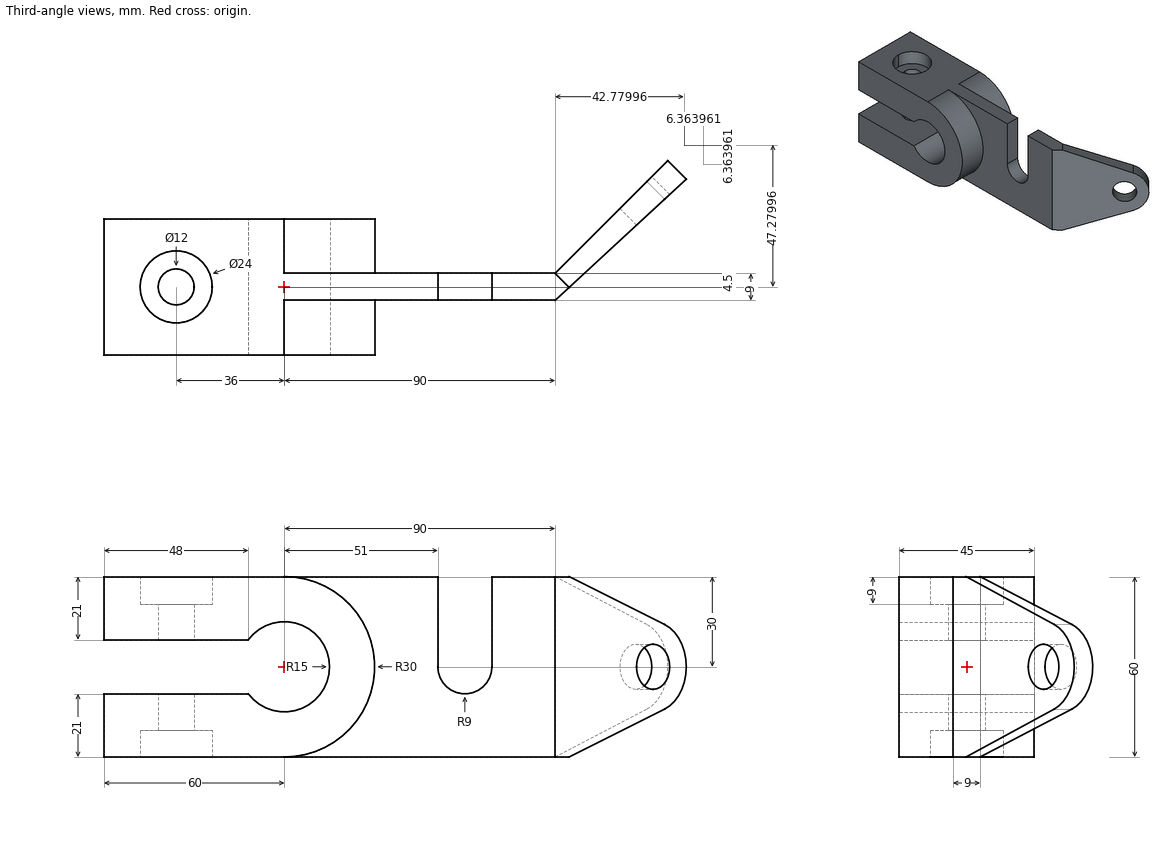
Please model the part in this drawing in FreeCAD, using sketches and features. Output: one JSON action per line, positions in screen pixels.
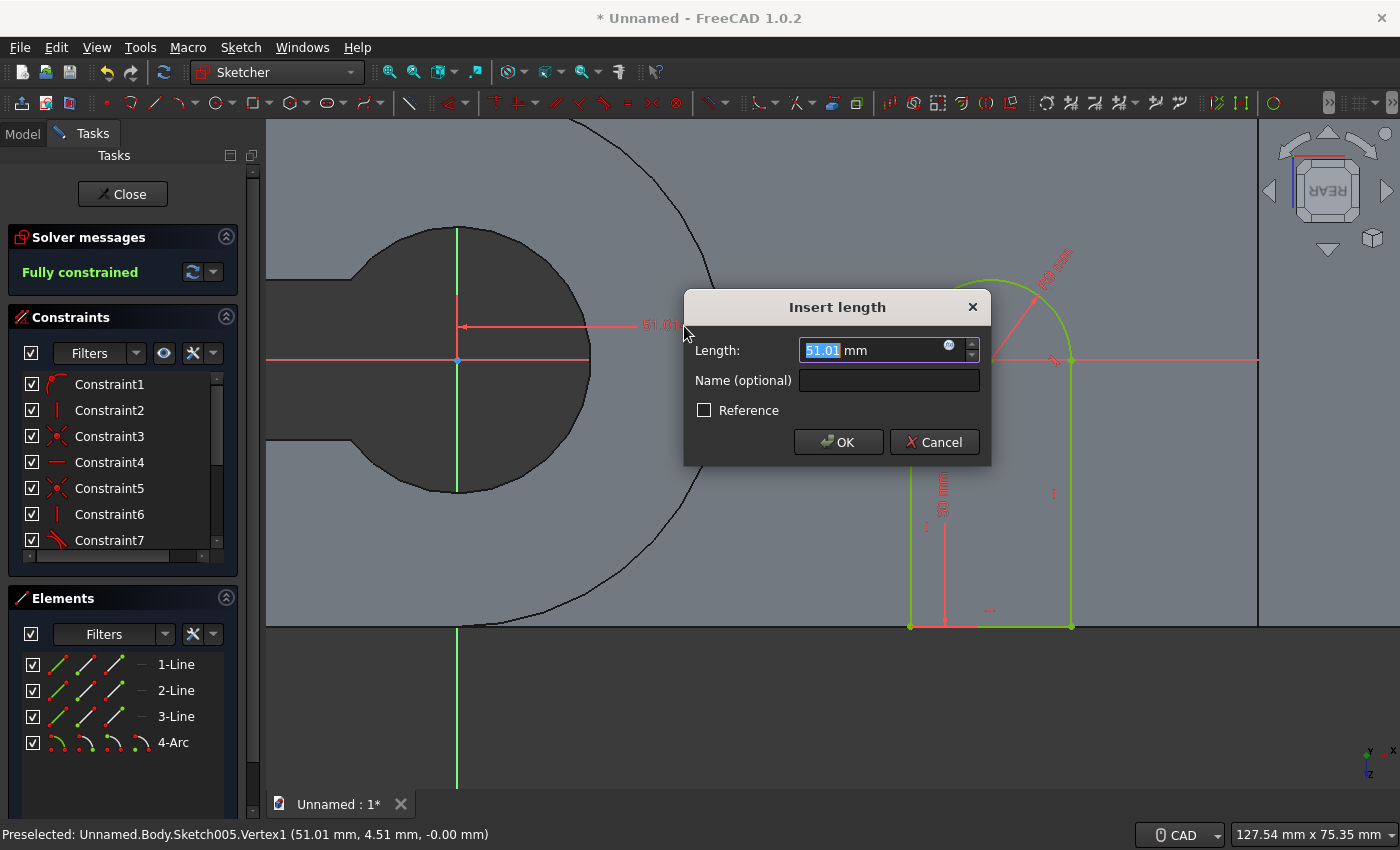
{"action": "type", "text": "51"}
{"action": "key", "text": "Return"}
{"action": "key", "text": "Escape"}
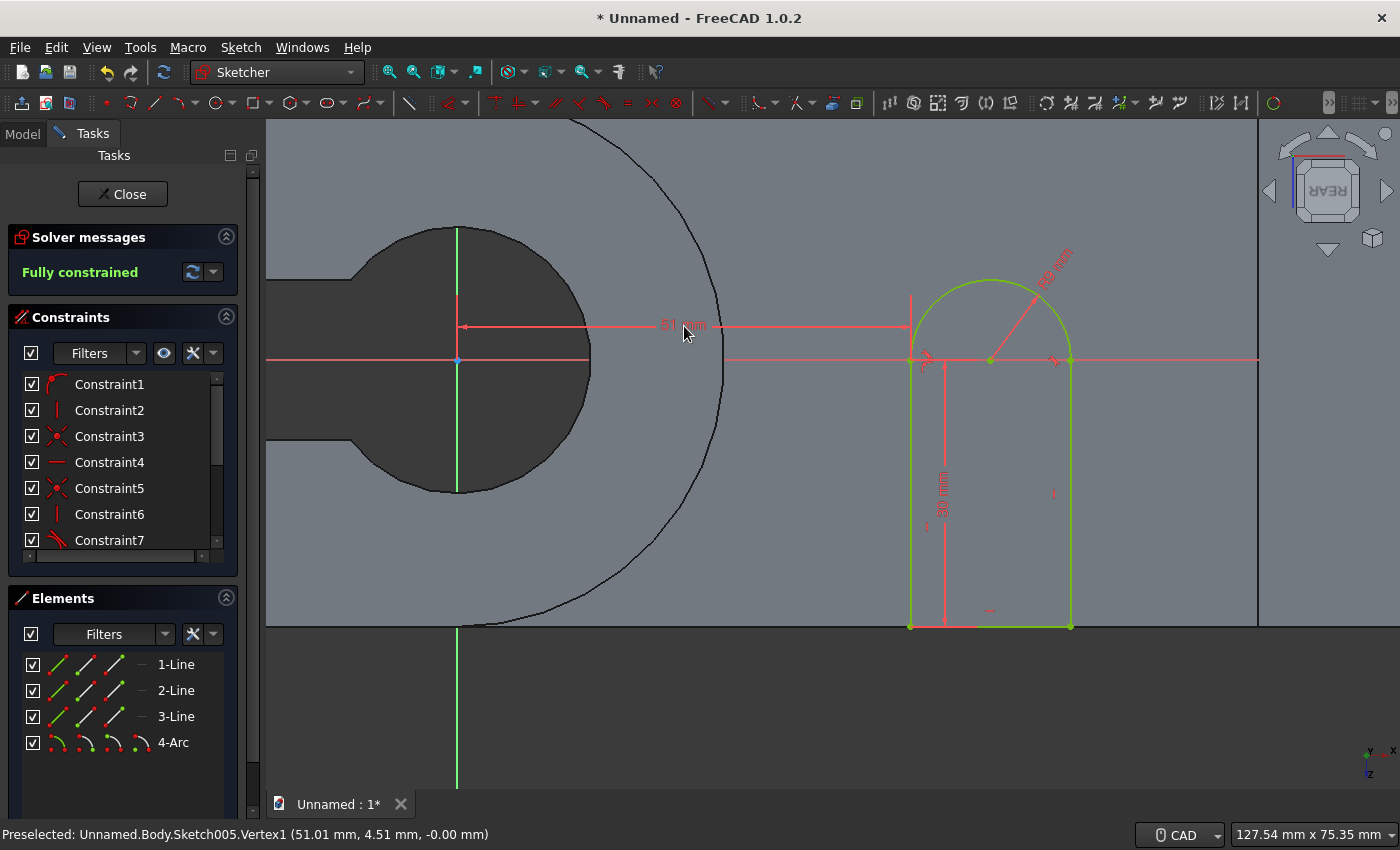
{"action": "left_click", "coordinate": [123, 194]}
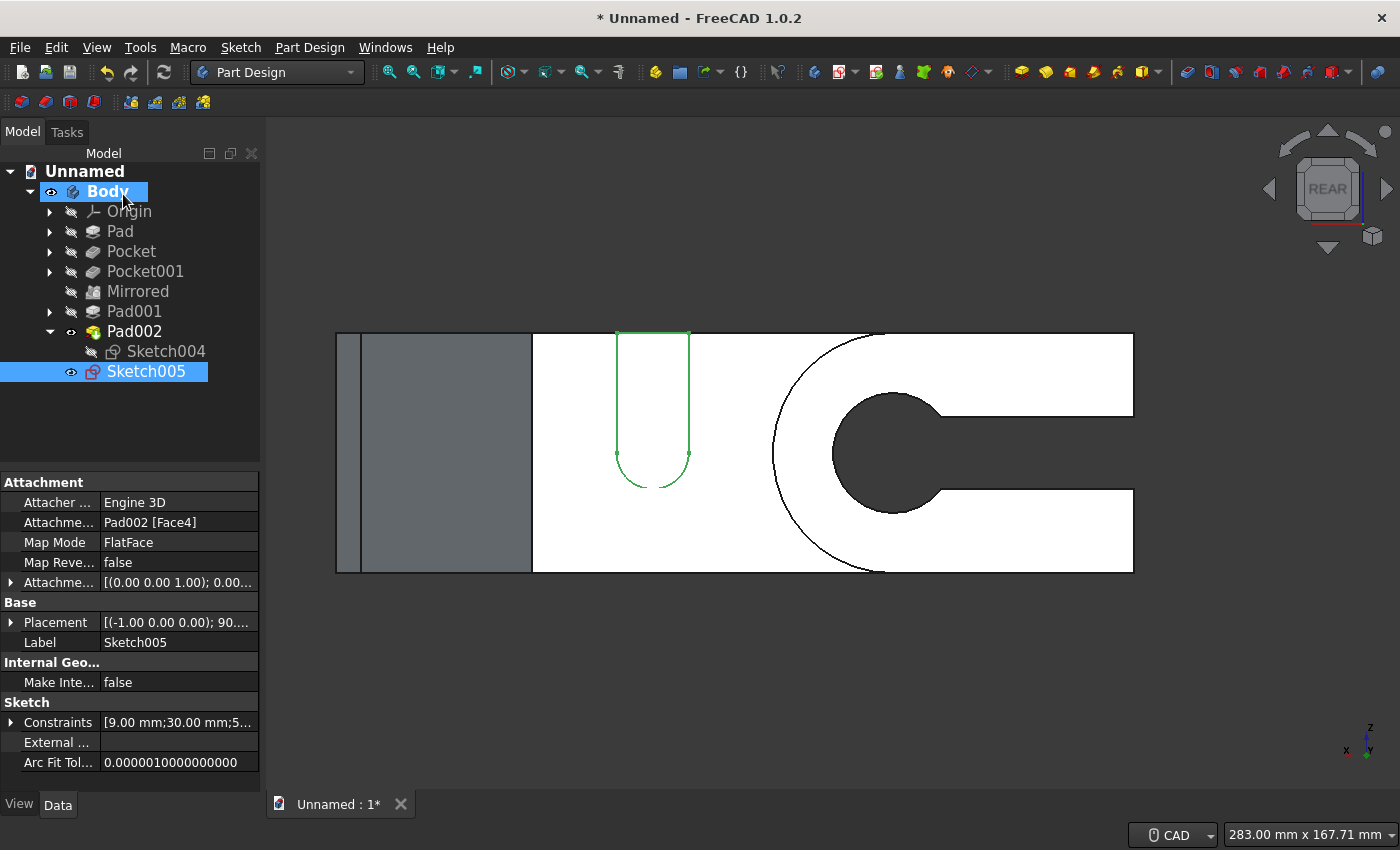
{"action": "left_click", "coordinate": [1188, 72]}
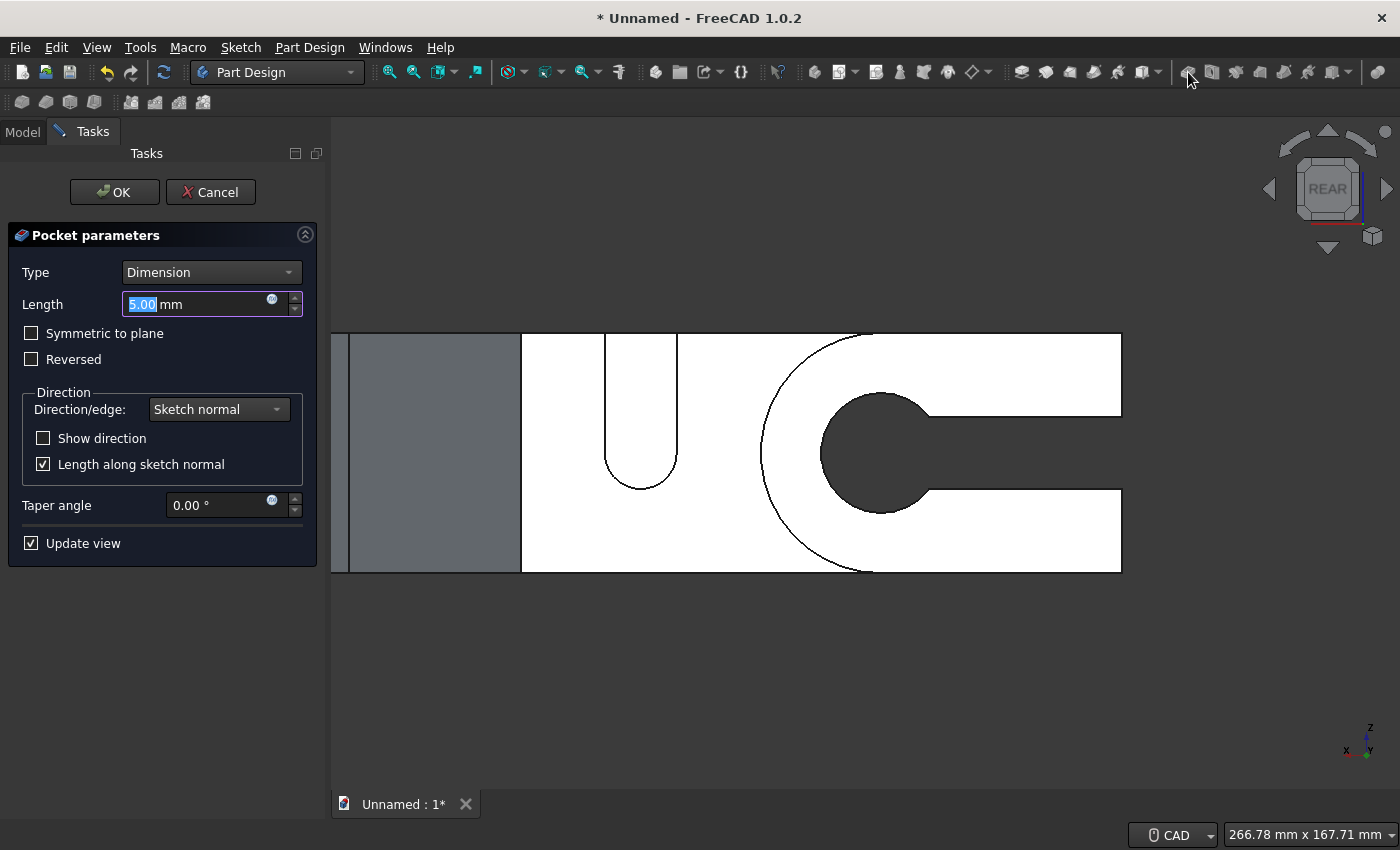
{"action": "type", "text": "9"}
{"action": "key", "text": "Tab"}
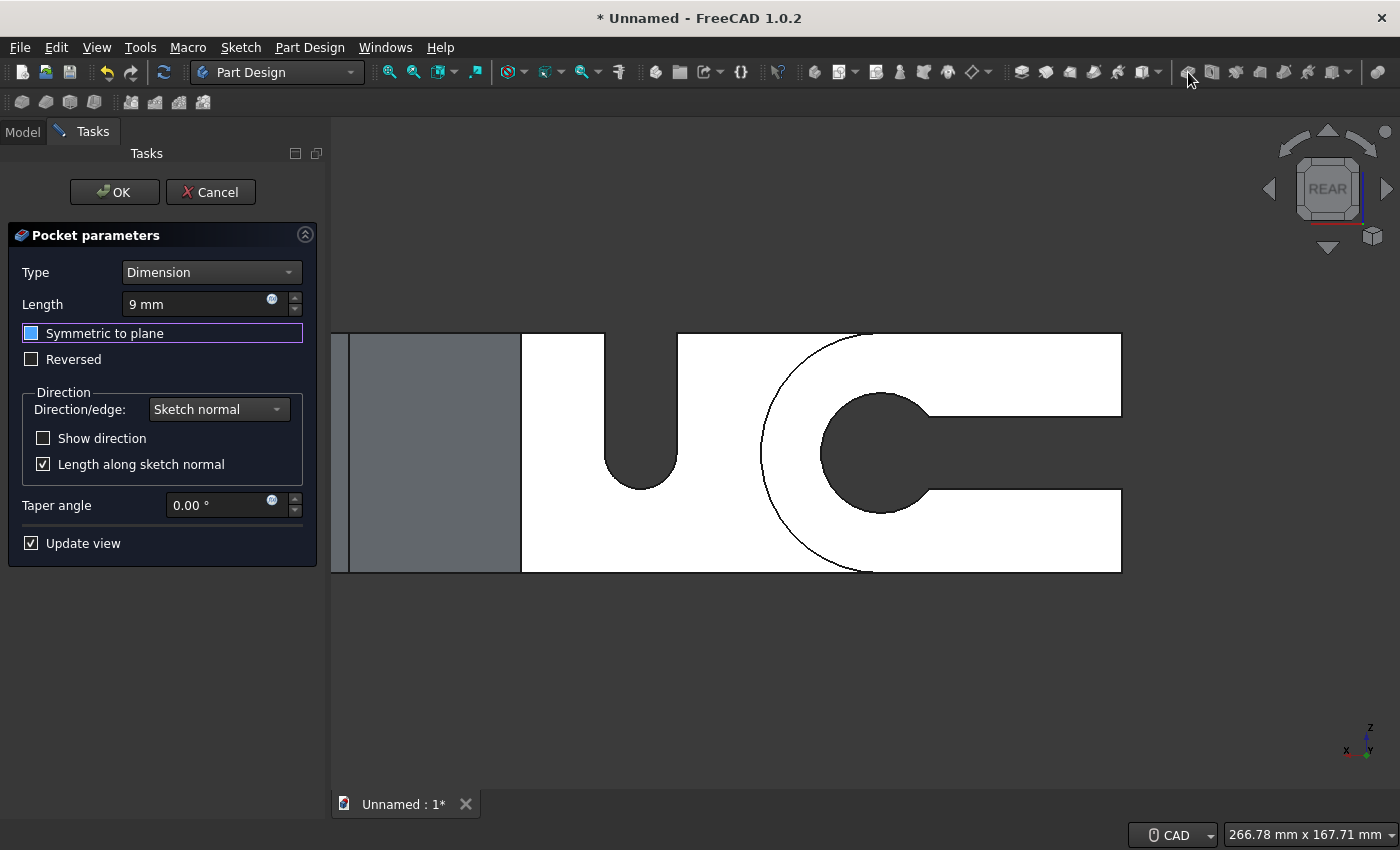
{"action": "left_click", "coordinate": [115, 192]}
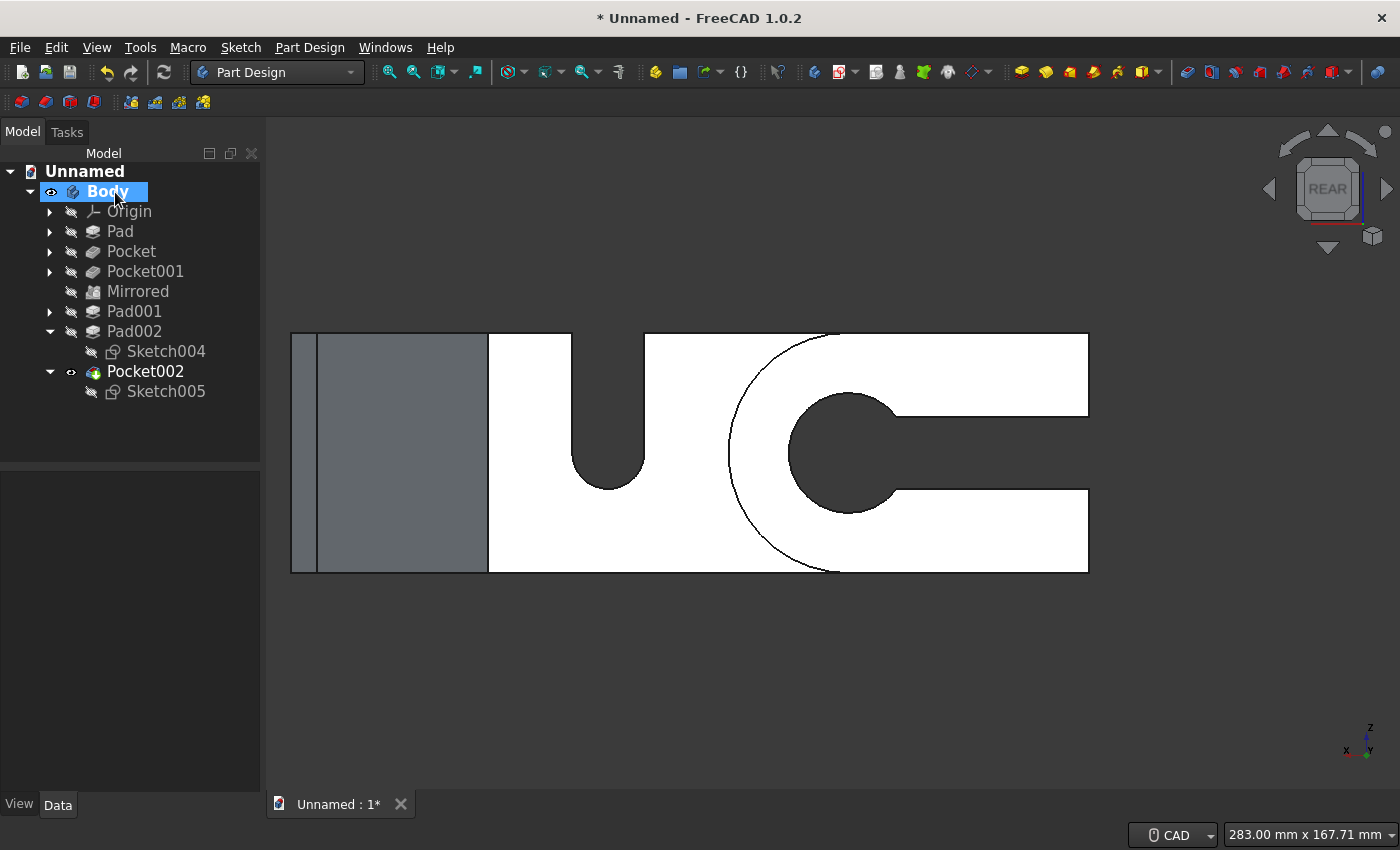
{"action": "left_click", "coordinate": [402, 452]}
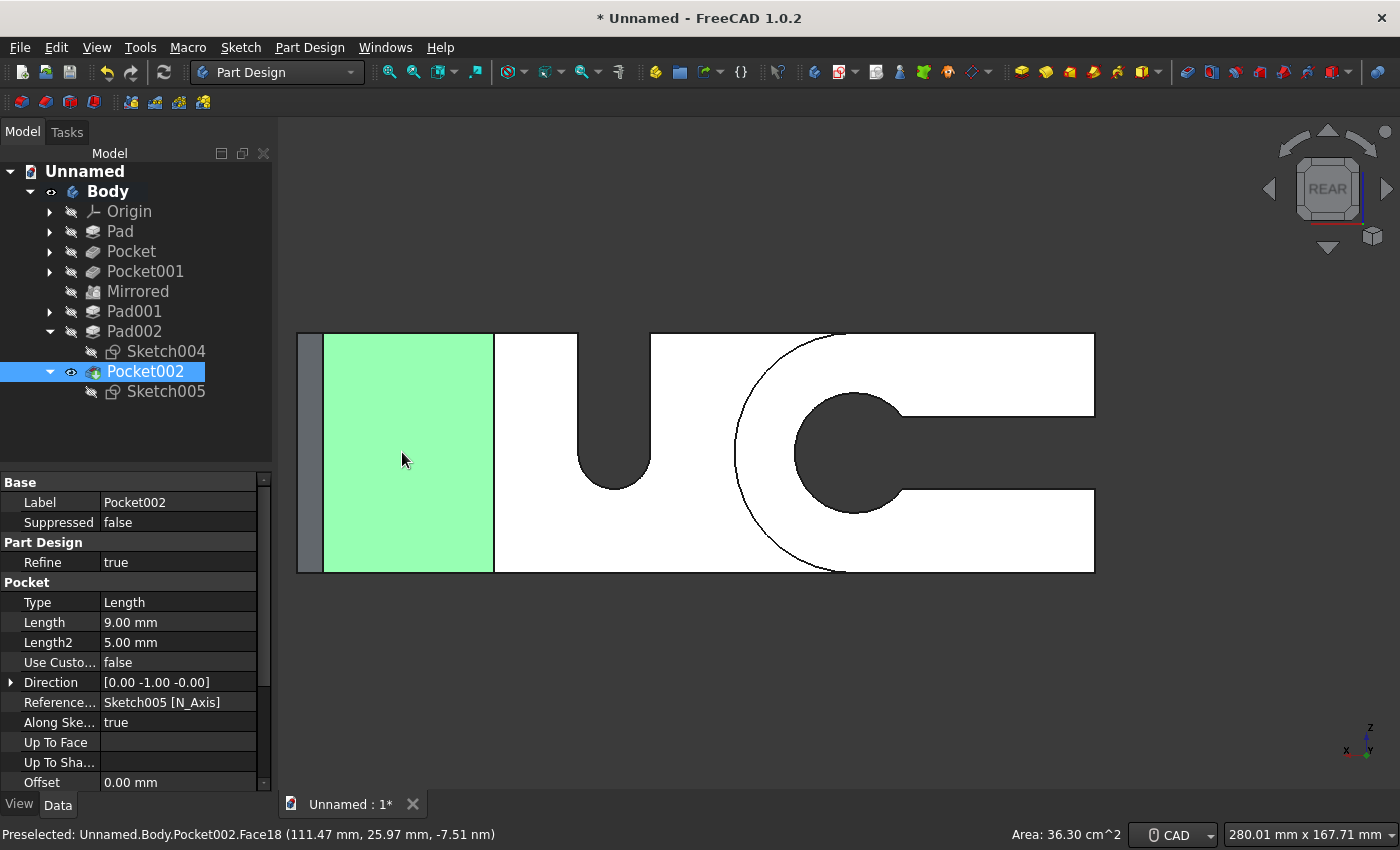
{"action": "left_click", "coordinate": [840, 72]}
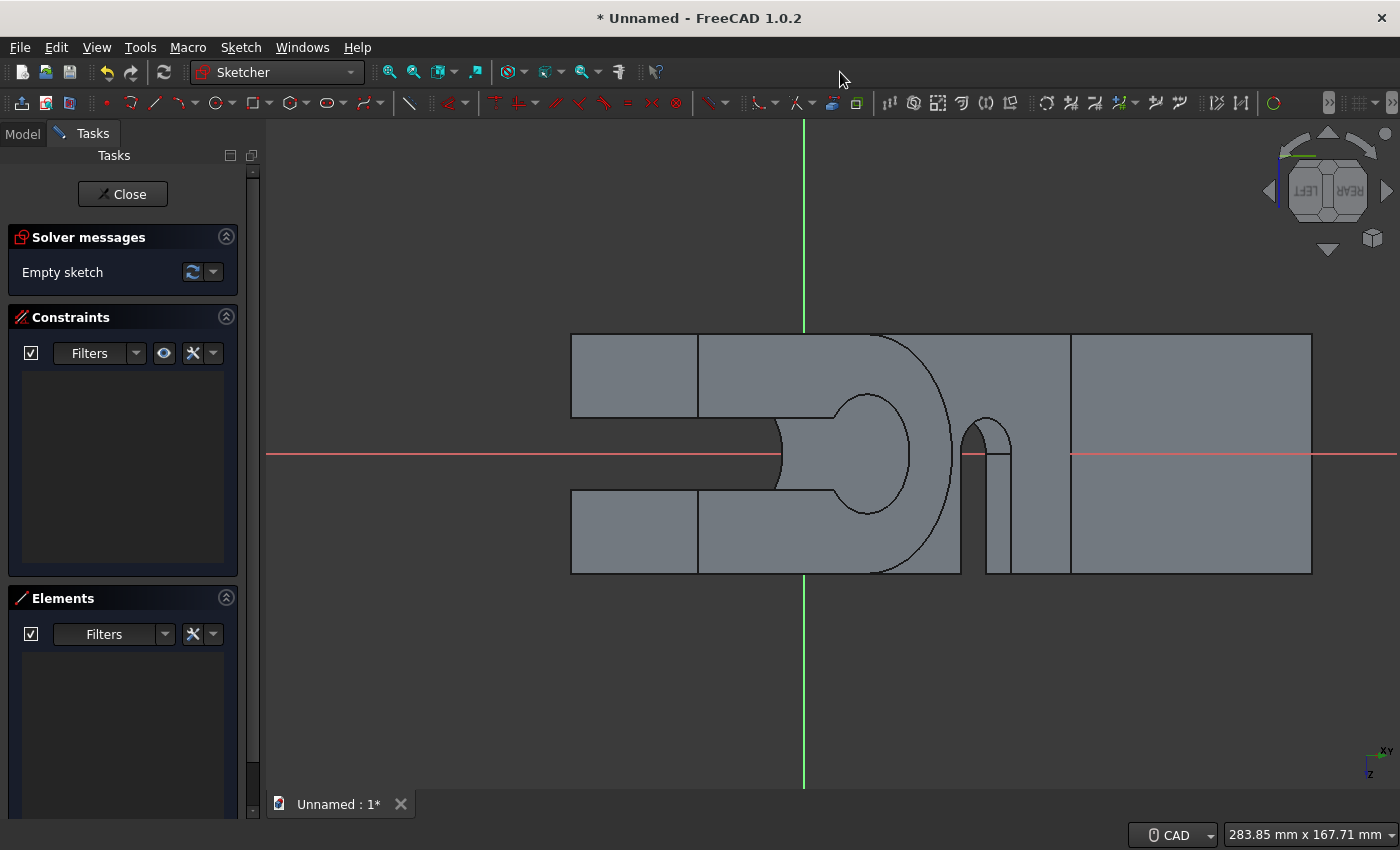
{"action": "key", "text": "q s"}